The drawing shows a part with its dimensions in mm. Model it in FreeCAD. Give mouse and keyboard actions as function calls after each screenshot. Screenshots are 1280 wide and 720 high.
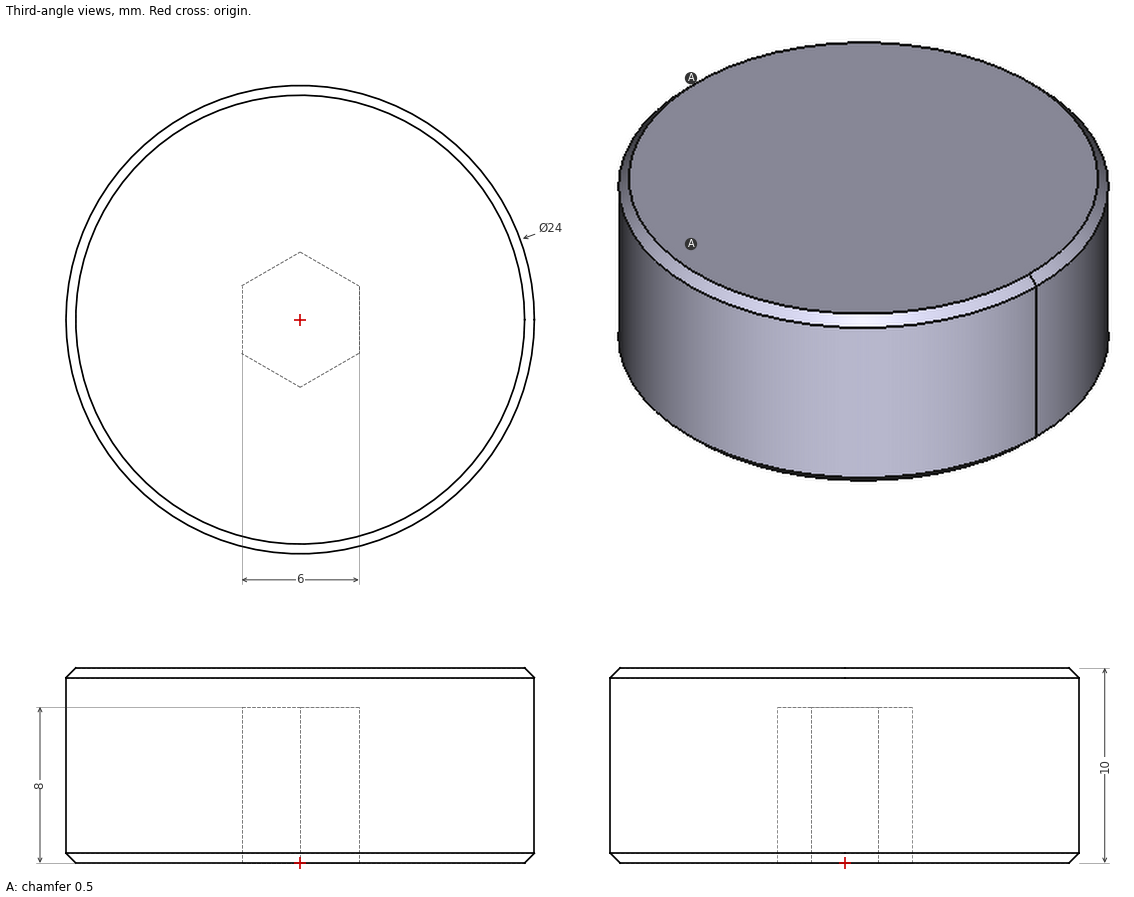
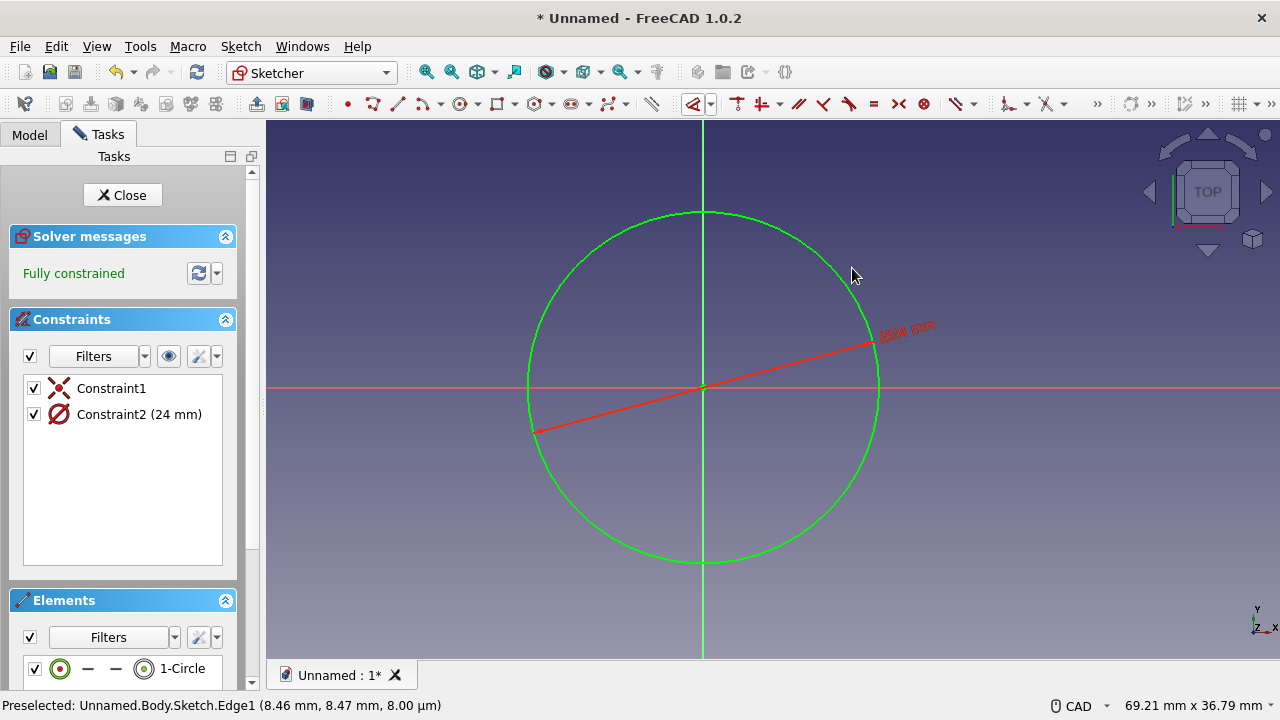
click(123, 195)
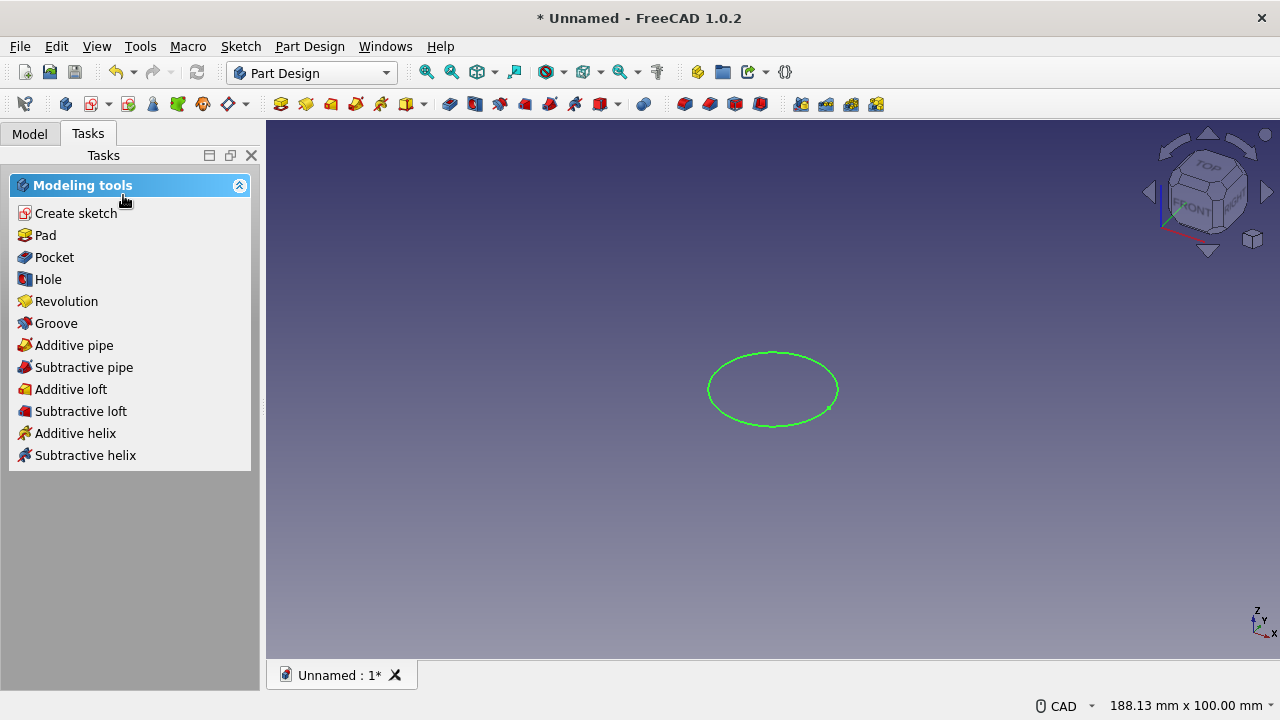
click(281, 104)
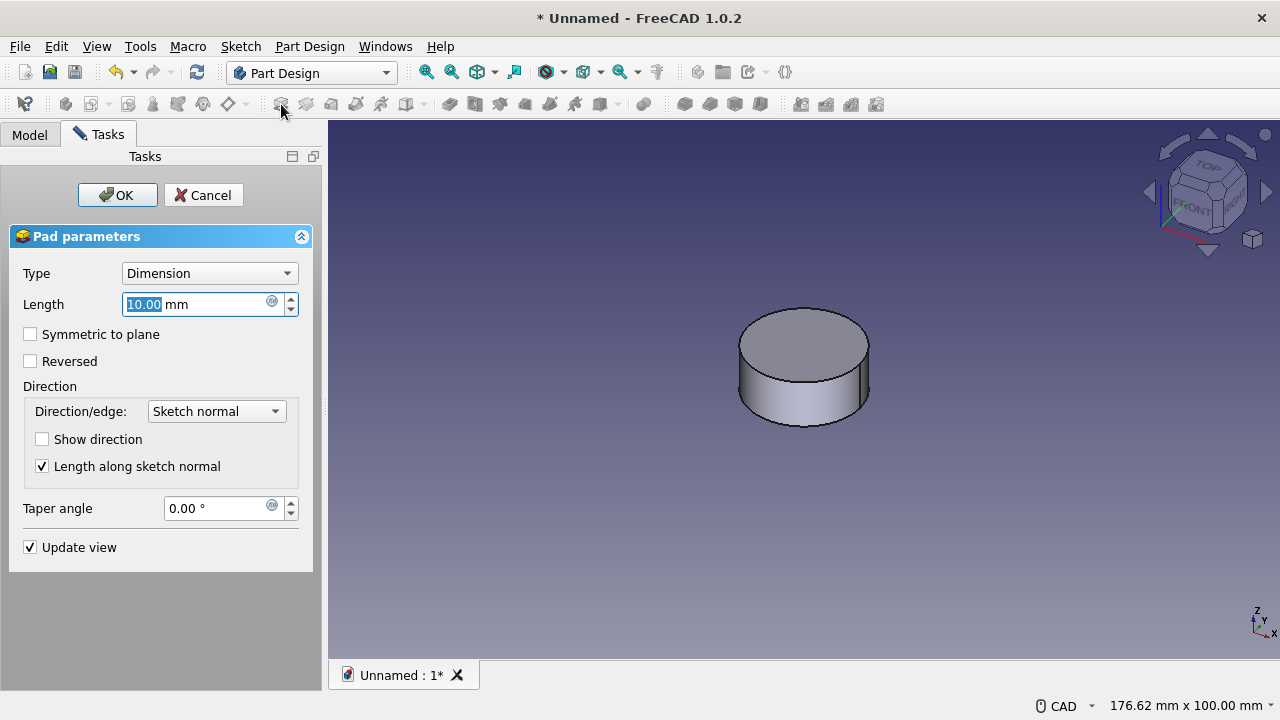
text(10)
key(Tab)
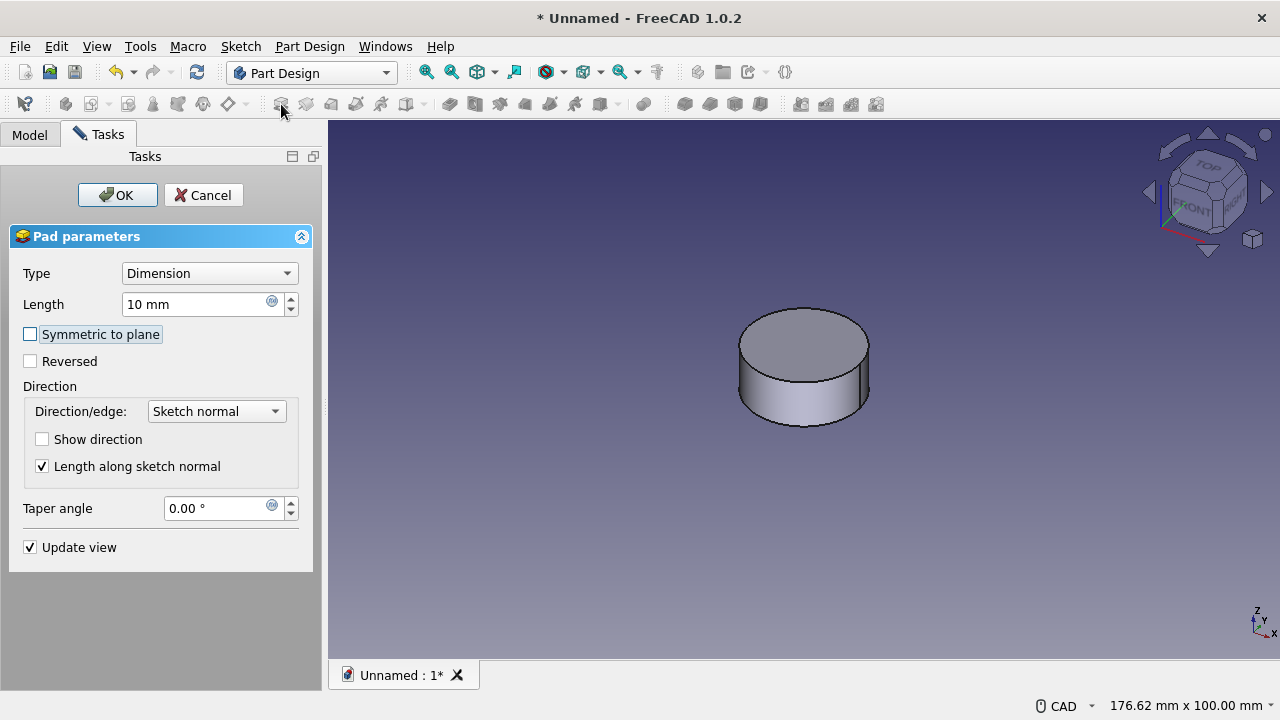
click(118, 195)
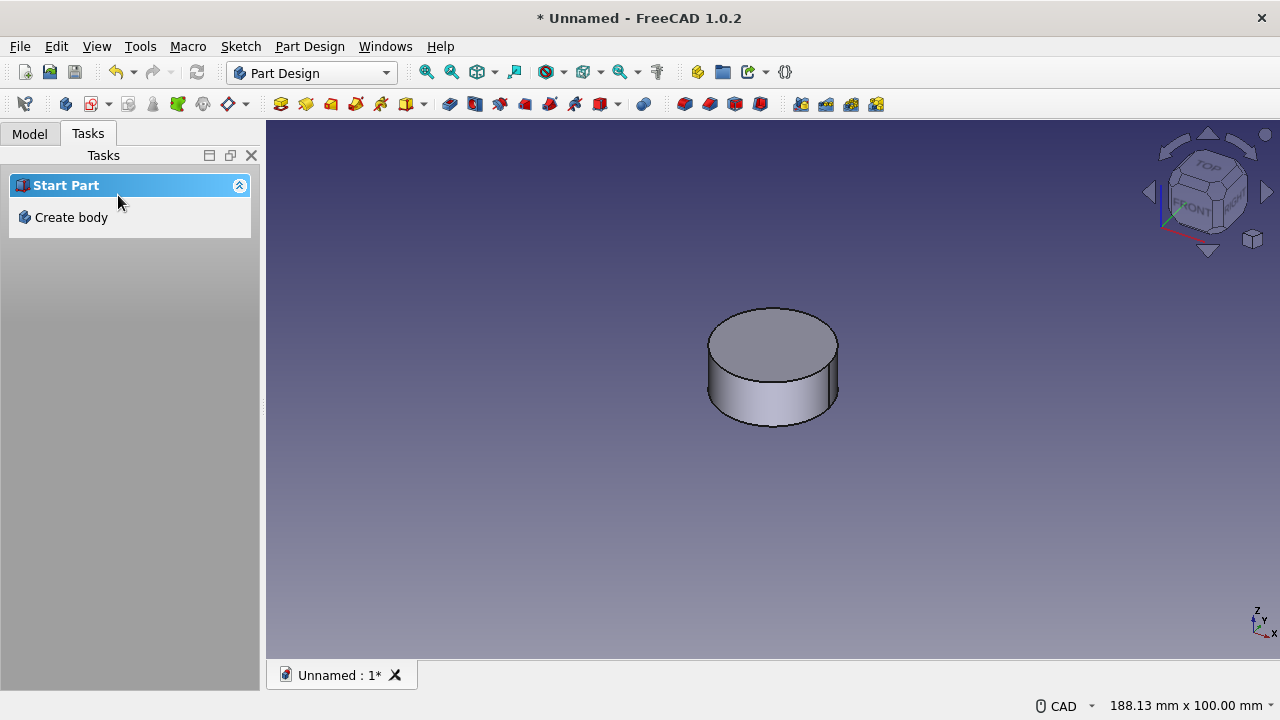
click(427, 72)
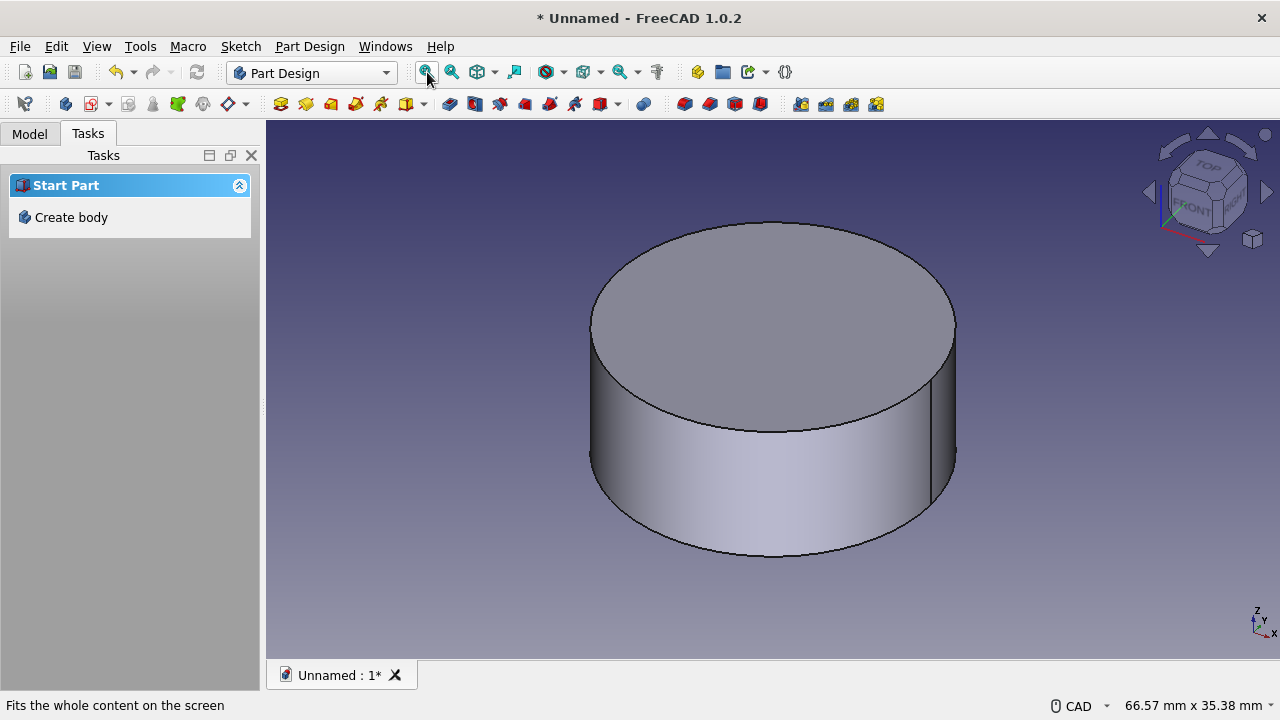
click(591, 337)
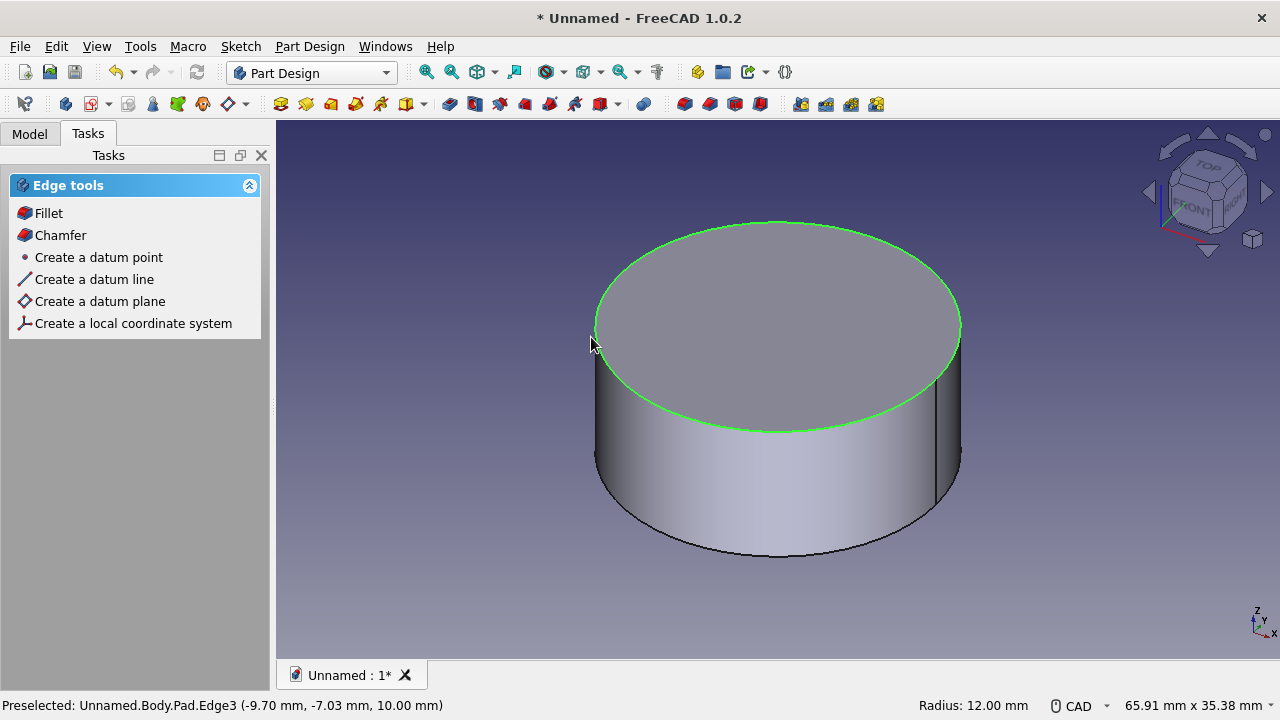
key(0)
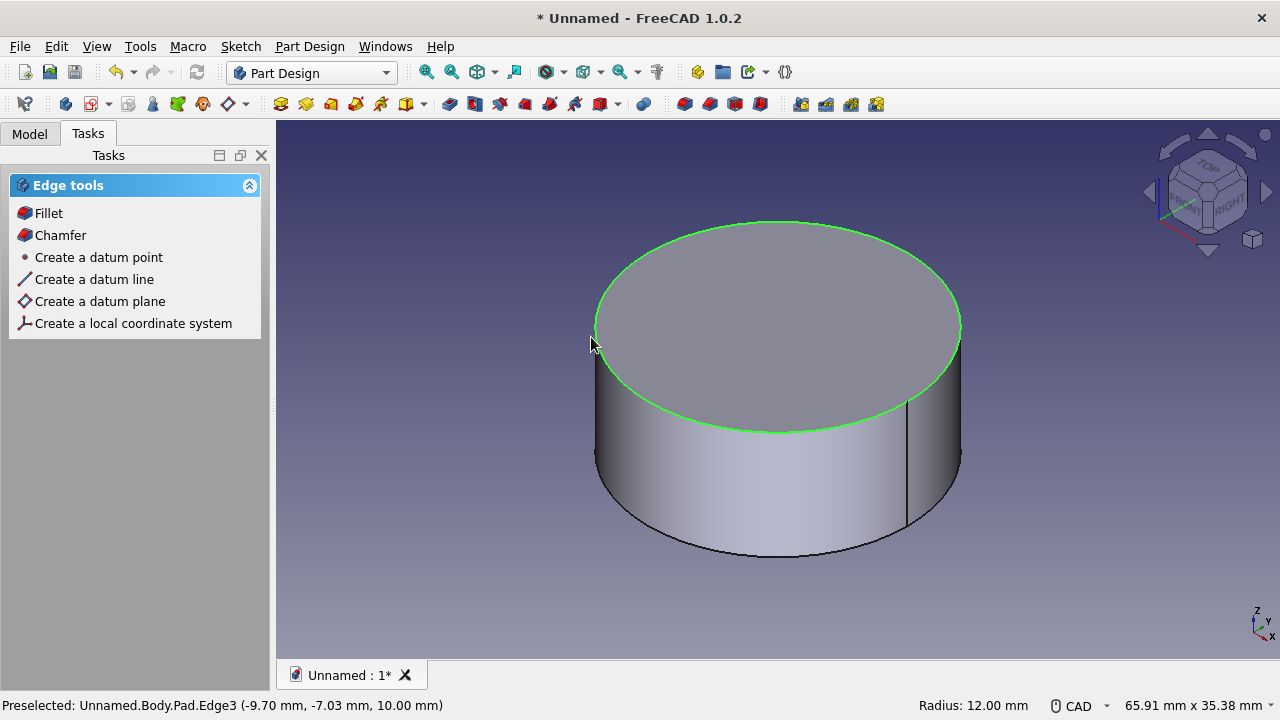
key(2)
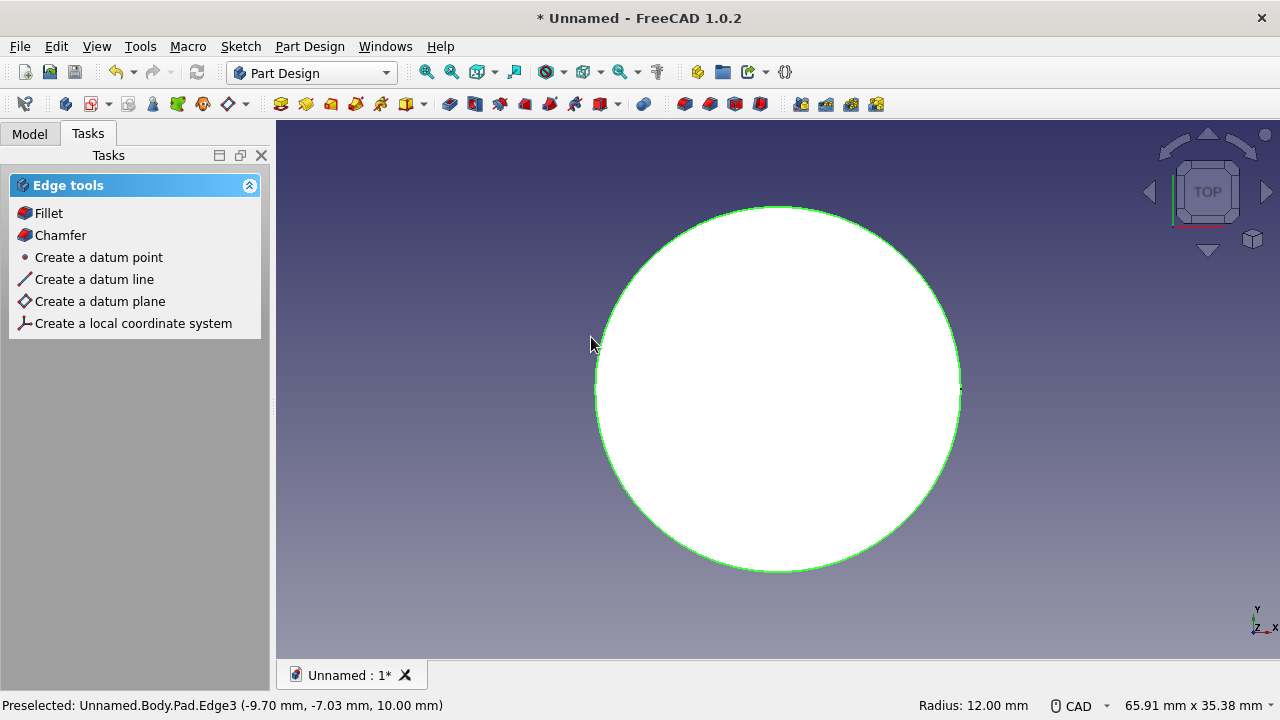
key(1)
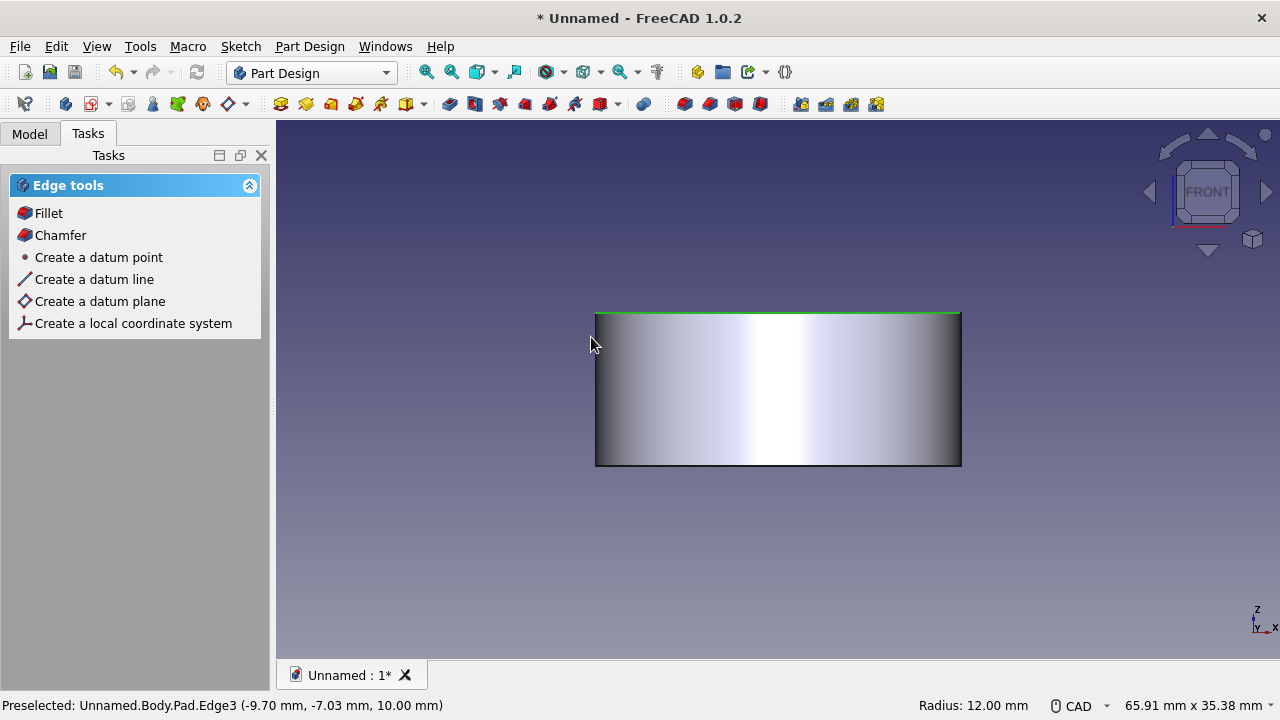
click(427, 72)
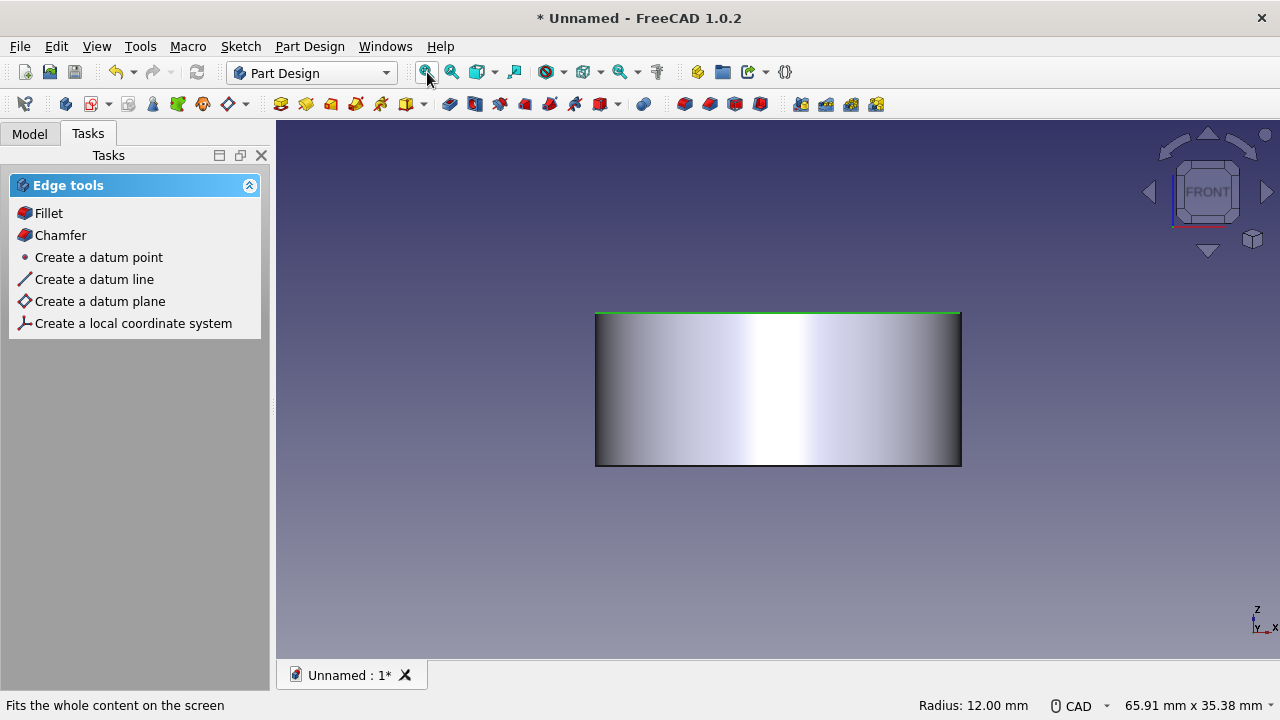
click(630, 465, ctrl)